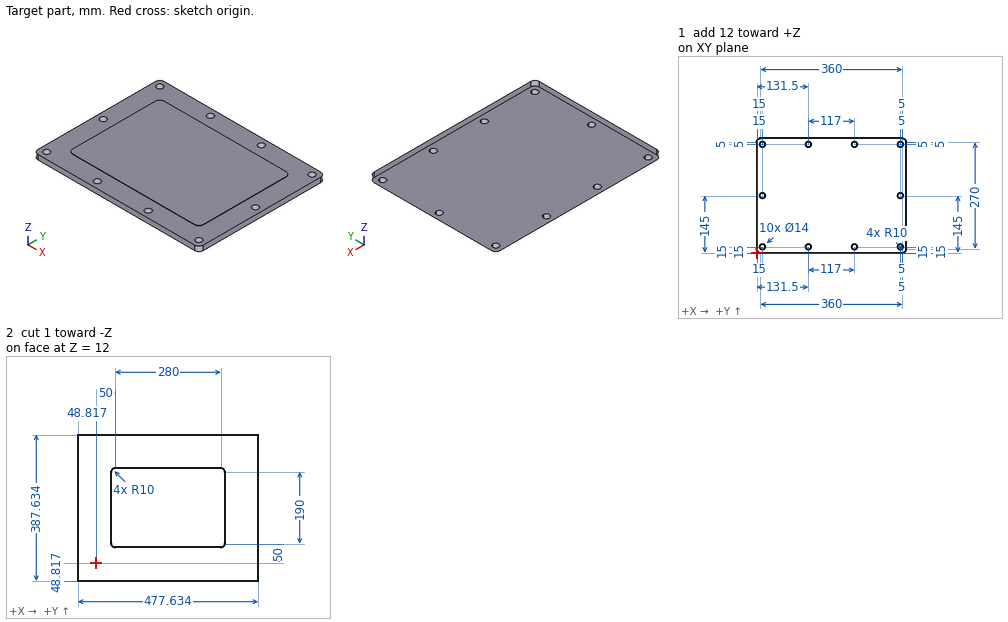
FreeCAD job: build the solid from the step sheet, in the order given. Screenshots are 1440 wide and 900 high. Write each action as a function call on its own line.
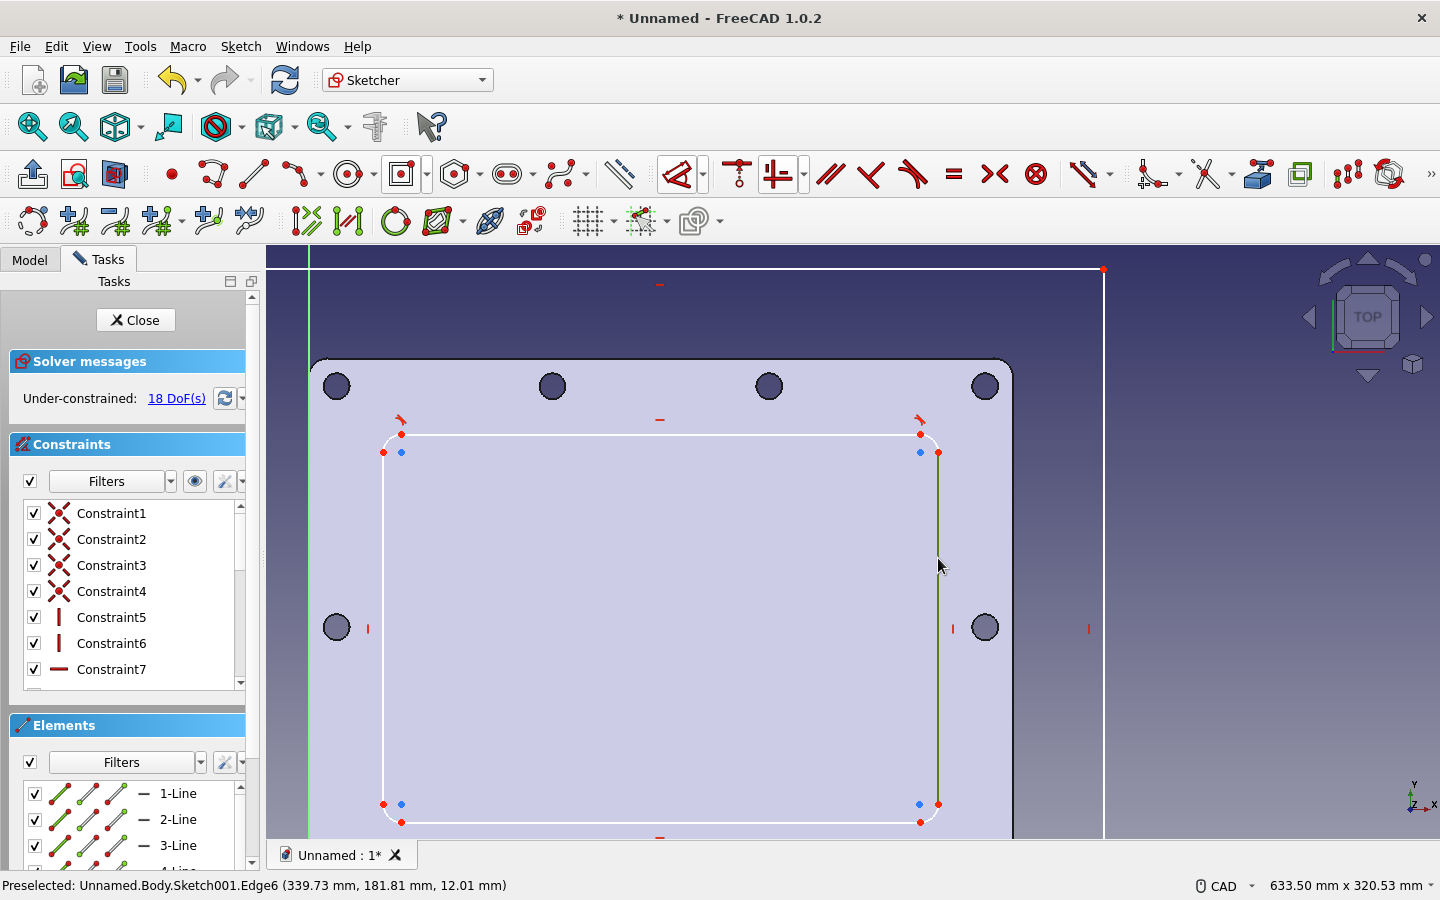
click(933, 440)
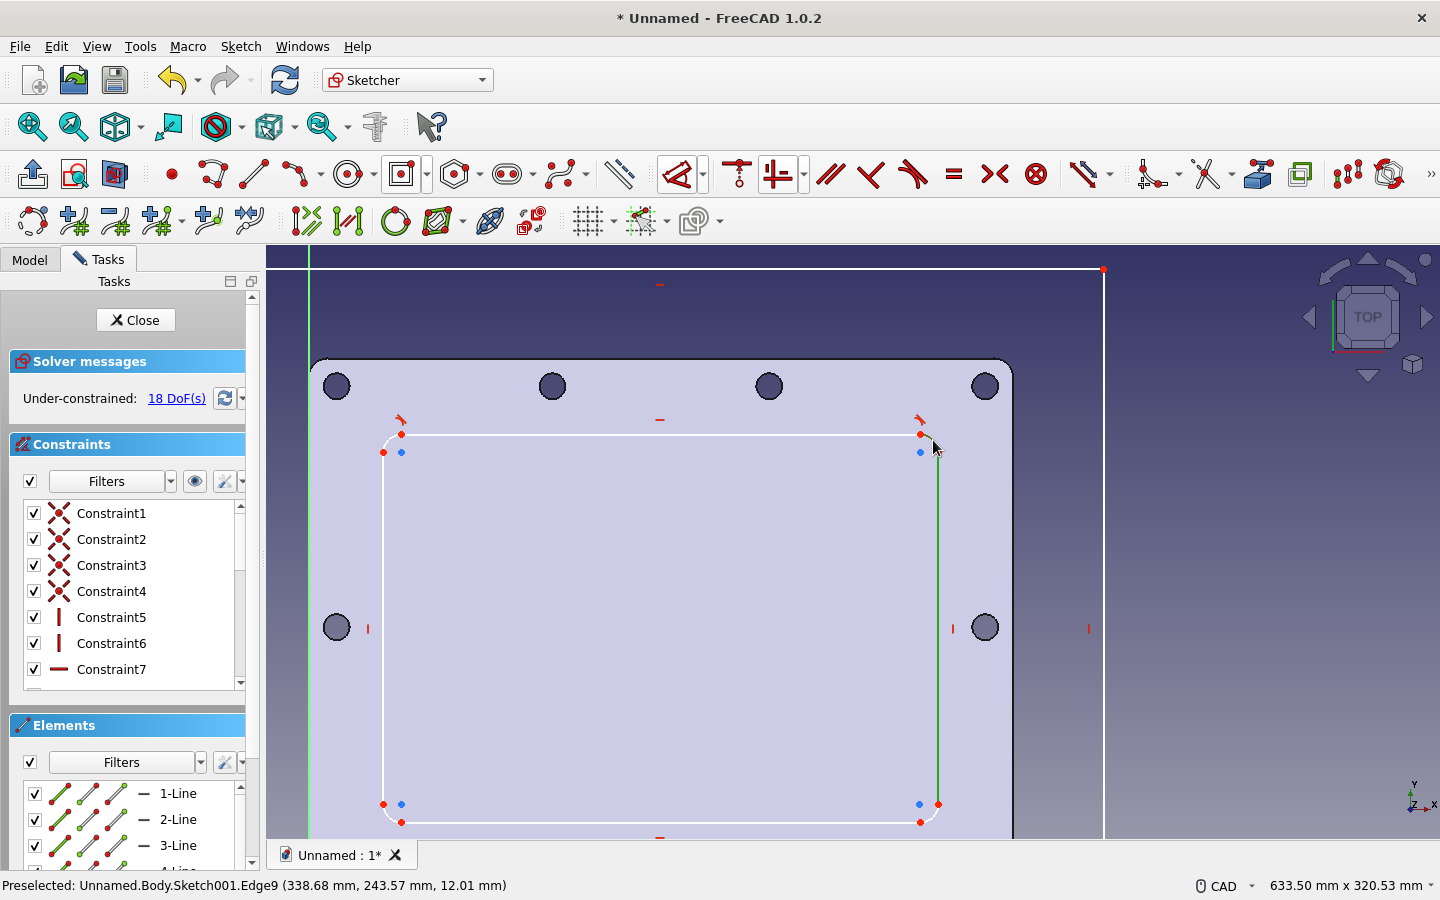
click(913, 174)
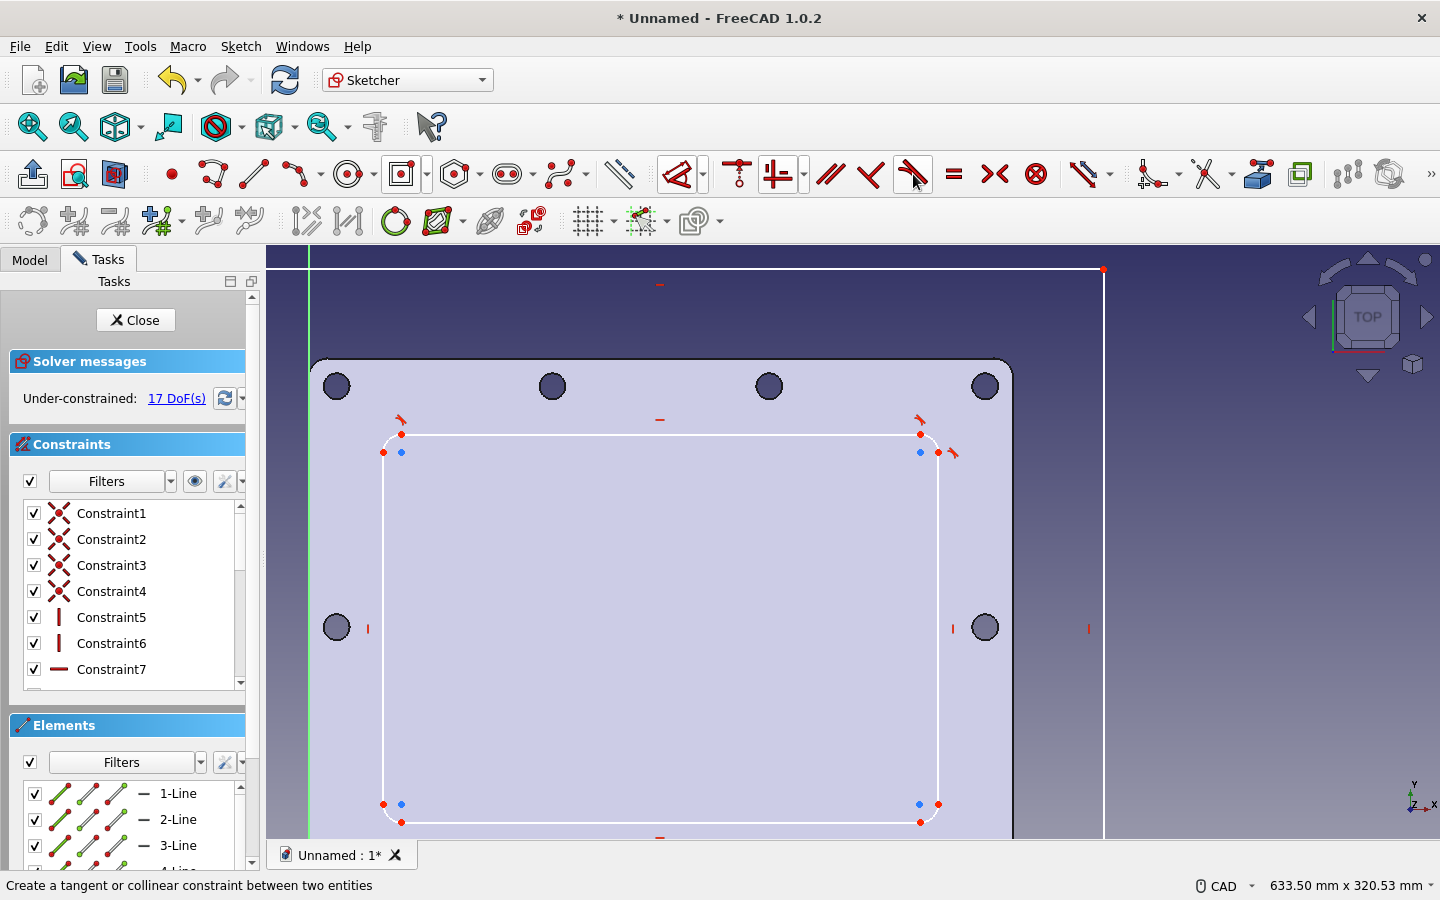
click(938, 558)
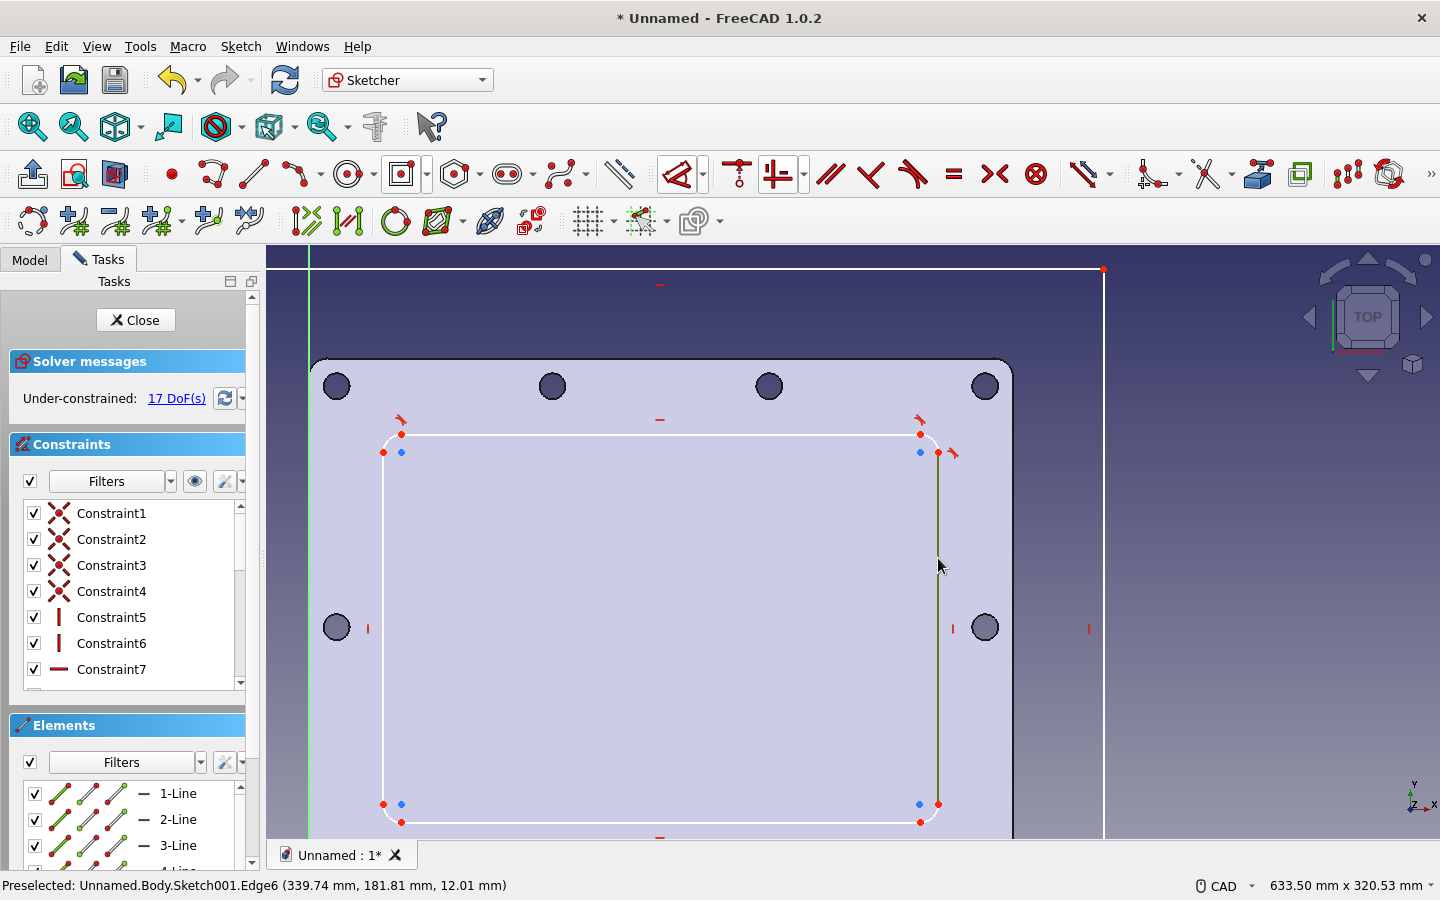
scroll(935, 438, down, 3)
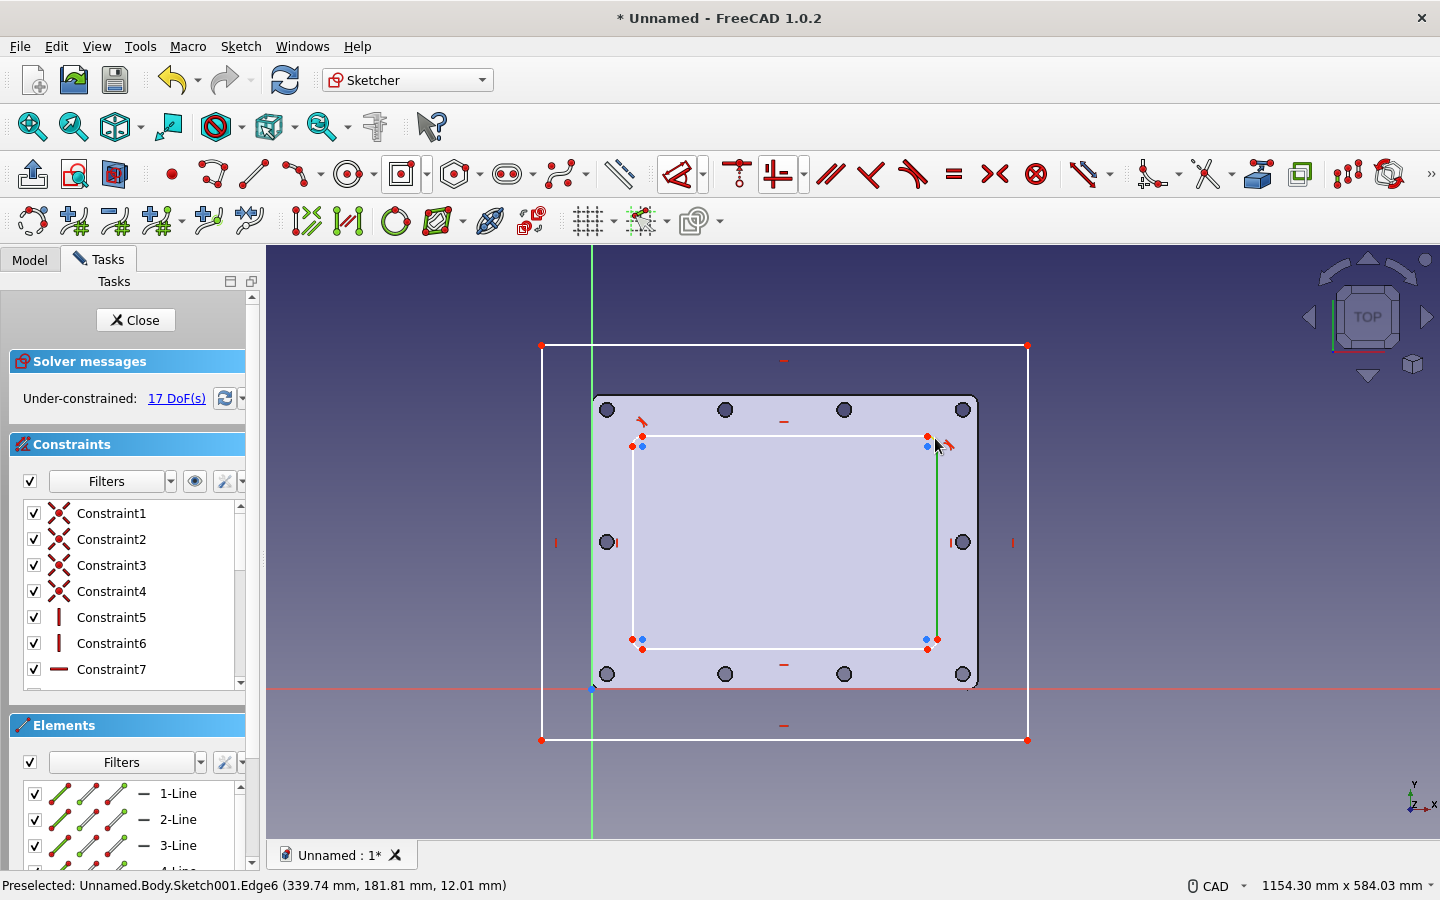
scroll(934, 646, up, 4)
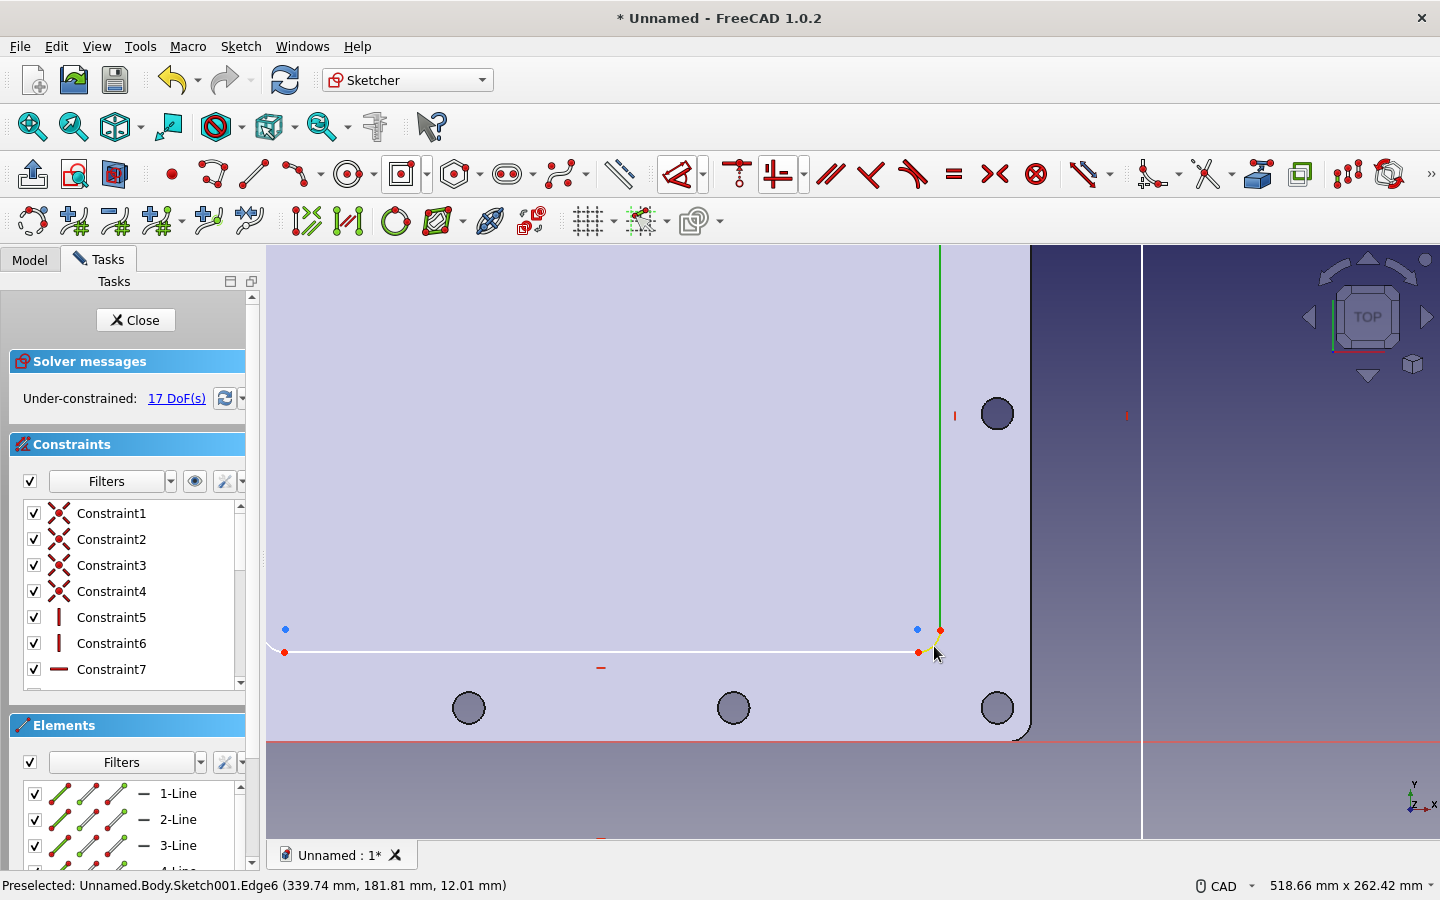
click(934, 646)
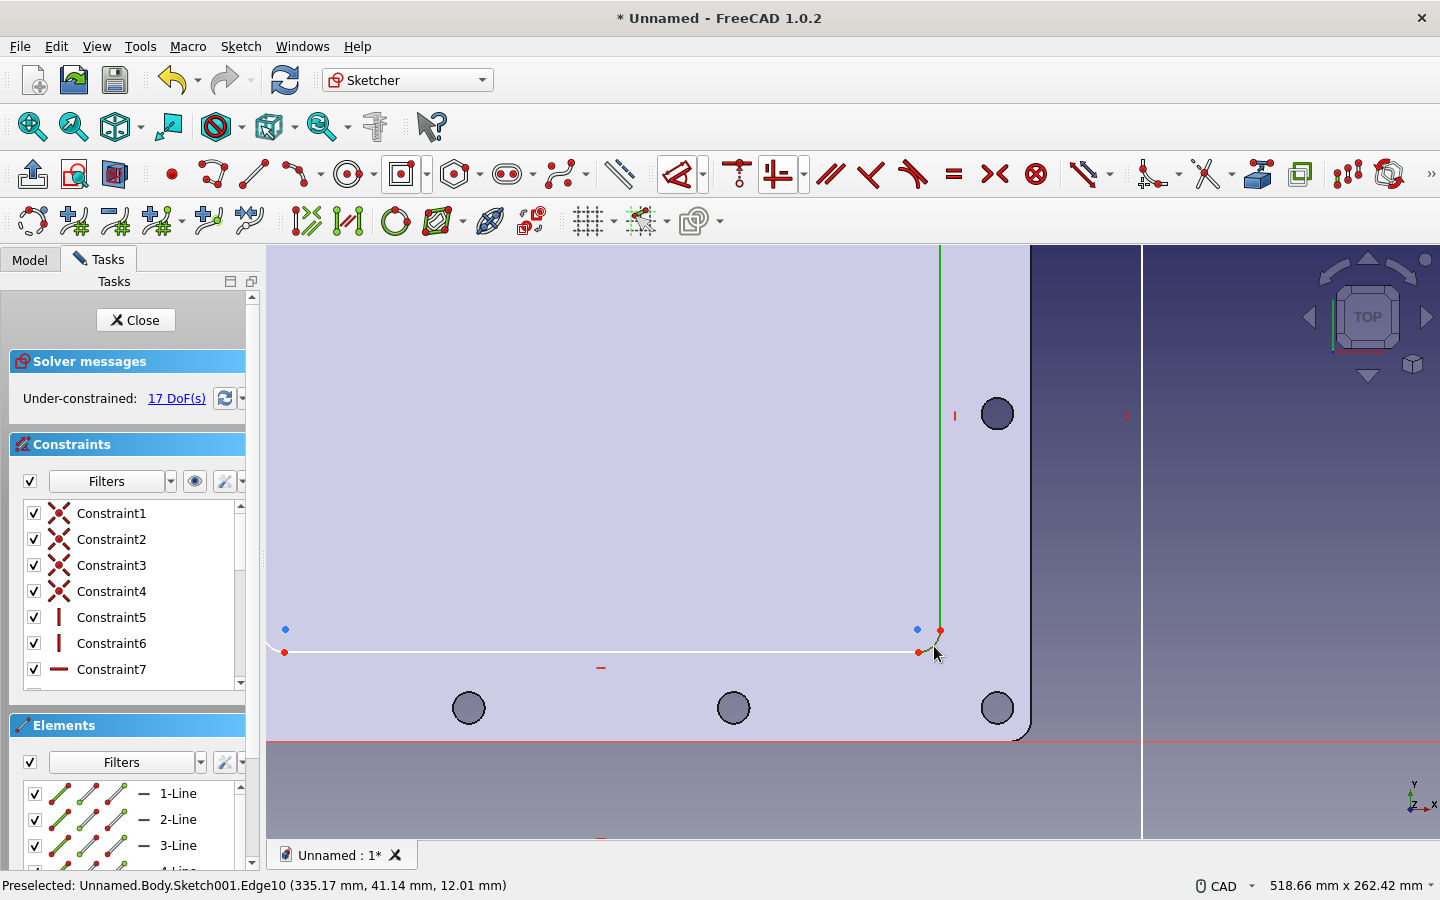
click(913, 174)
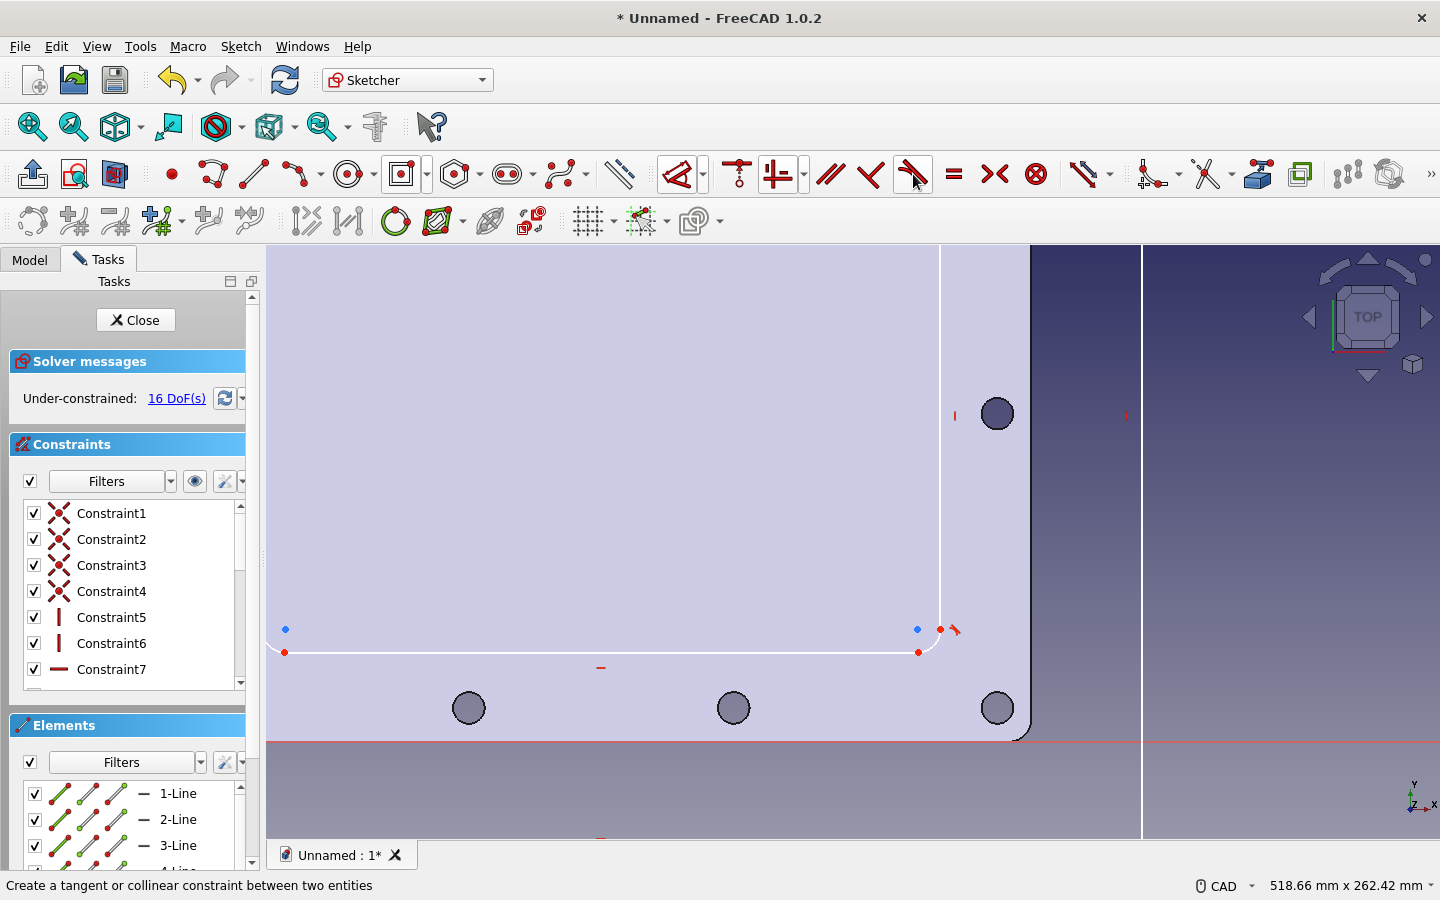
click(728, 653)